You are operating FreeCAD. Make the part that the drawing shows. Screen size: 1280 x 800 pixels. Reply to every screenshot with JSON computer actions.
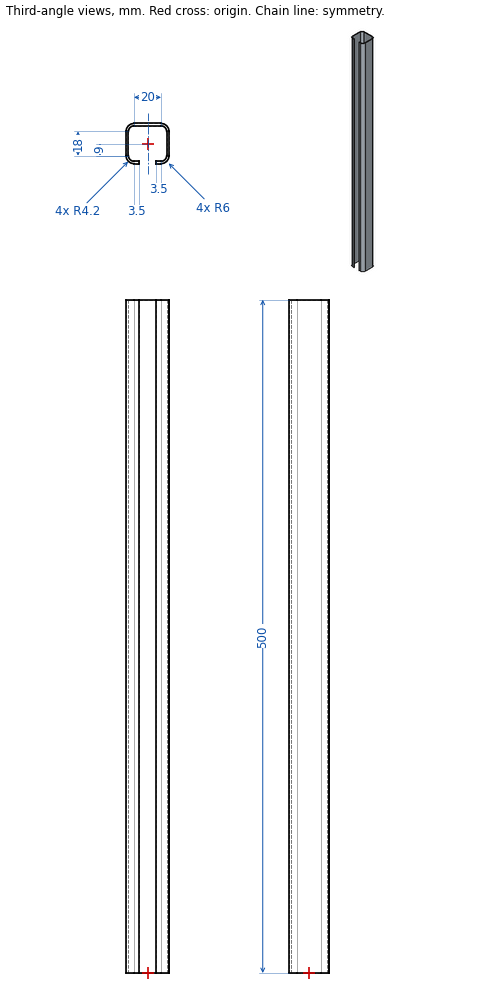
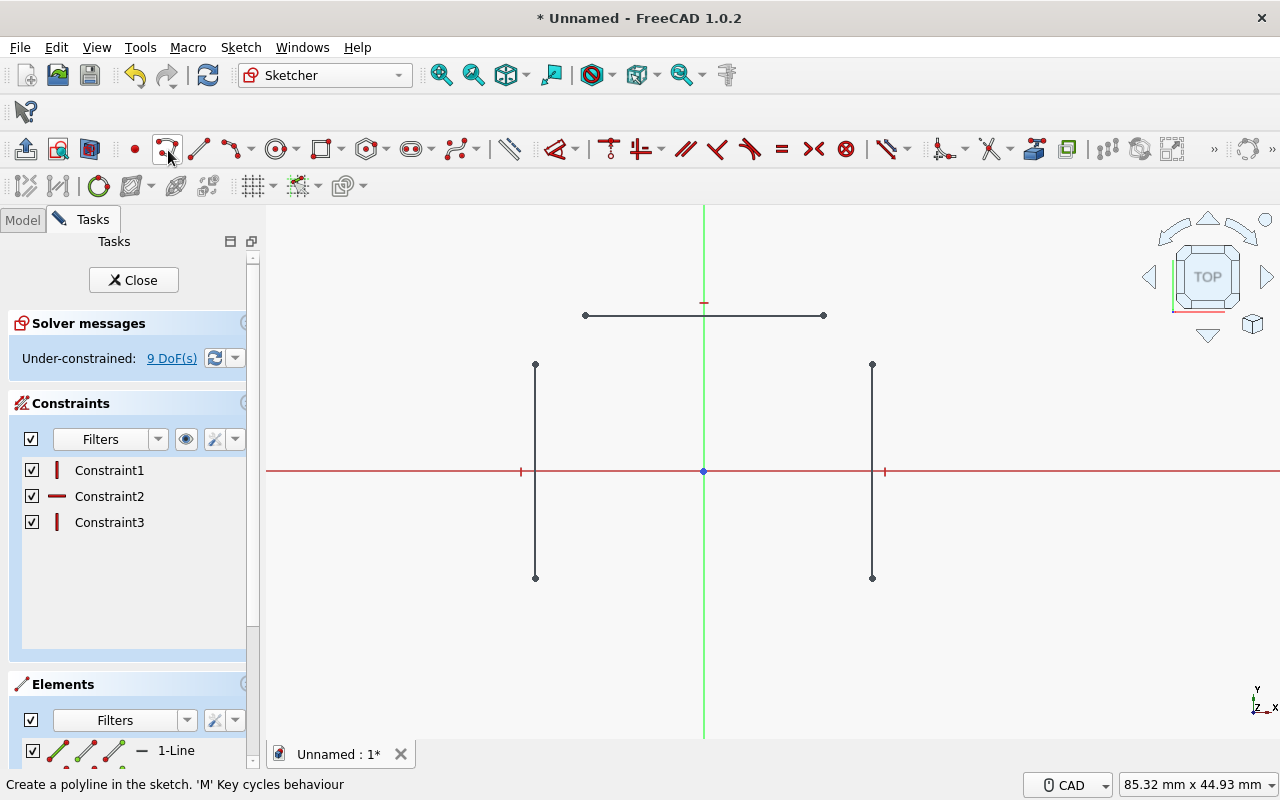
{"action": "left_click", "coordinate": [823, 628]}
{"action": "left_click", "coordinate": [781, 628]}
{"action": "left_click", "coordinate": [781, 650]}
{"action": "left_click", "coordinate": [823, 650]}
{"action": "right_click", "coordinate": [823, 650]}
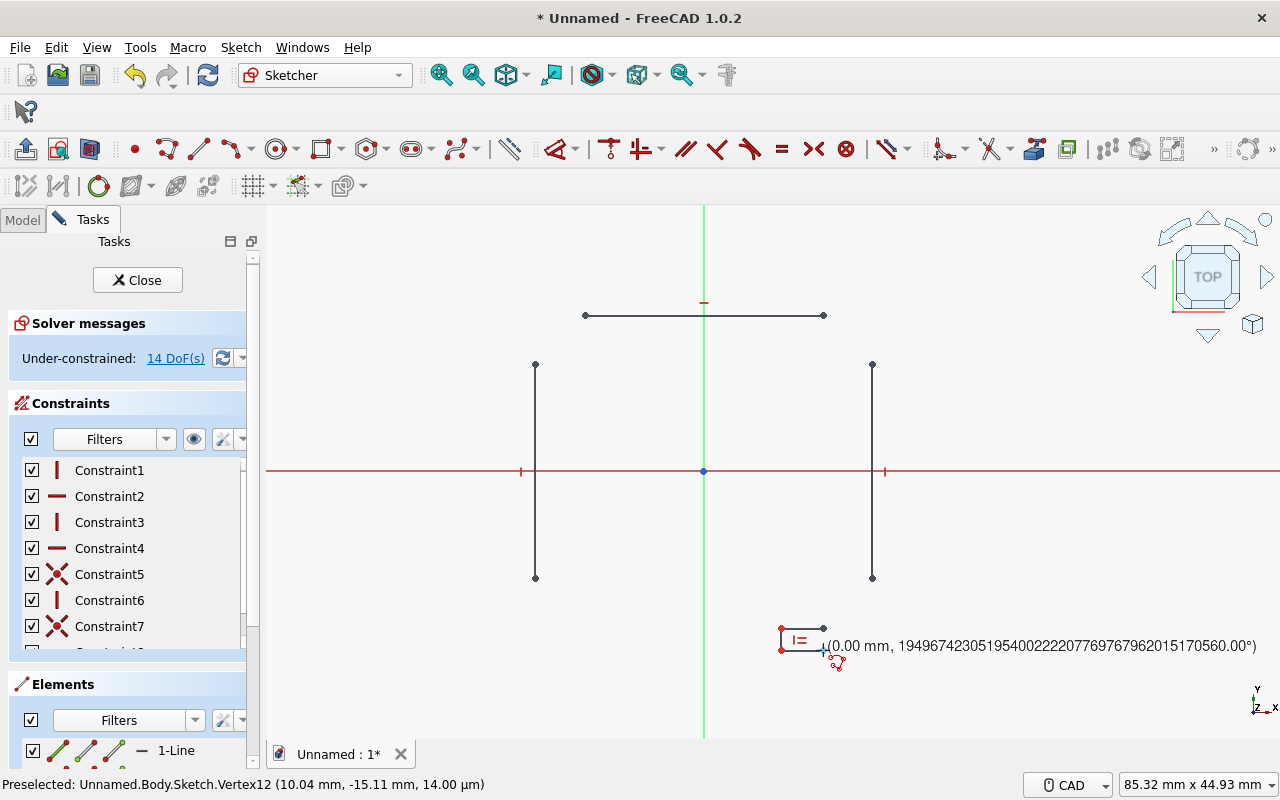
{"action": "left_click", "coordinate": [200, 150]}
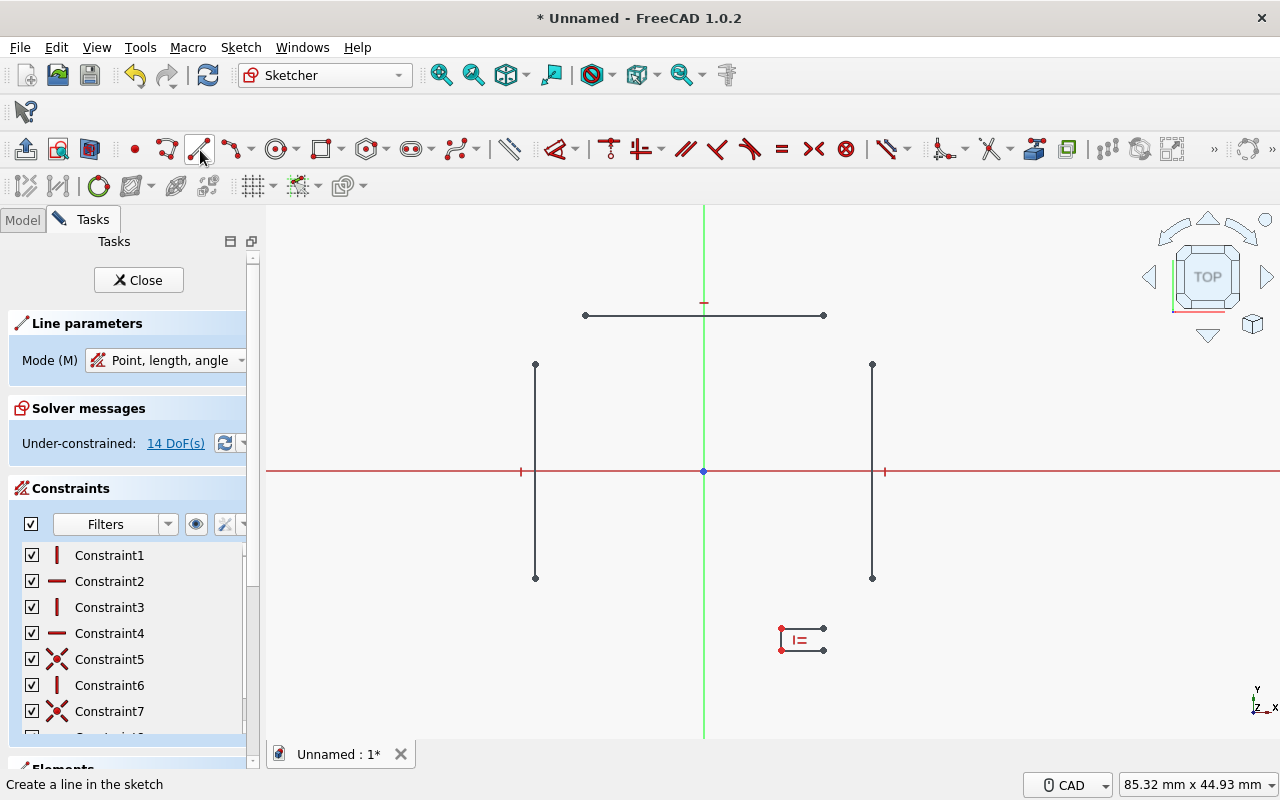
{"action": "left_click", "coordinate": [894, 578]}
{"action": "left_click", "coordinate": [894, 364]}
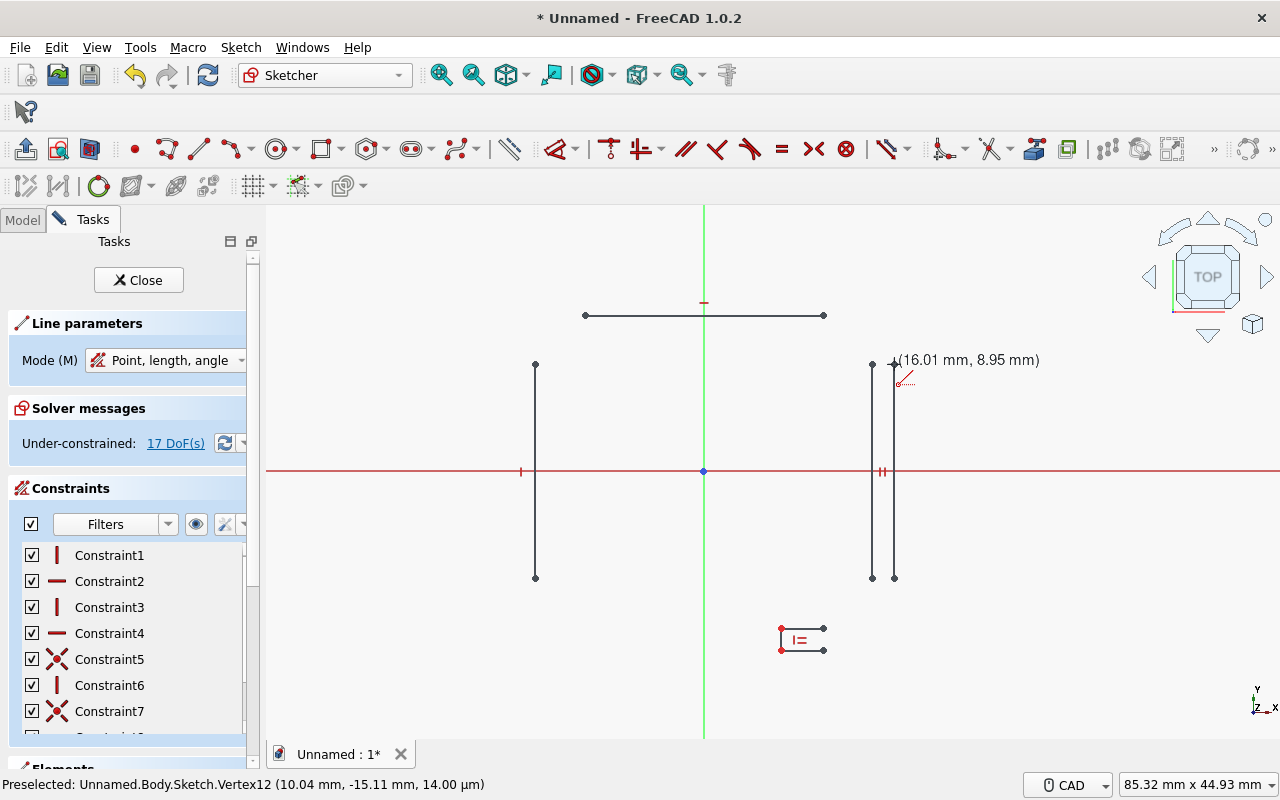
{"action": "left_click", "coordinate": [823, 293]}
{"action": "left_click", "coordinate": [585, 293]}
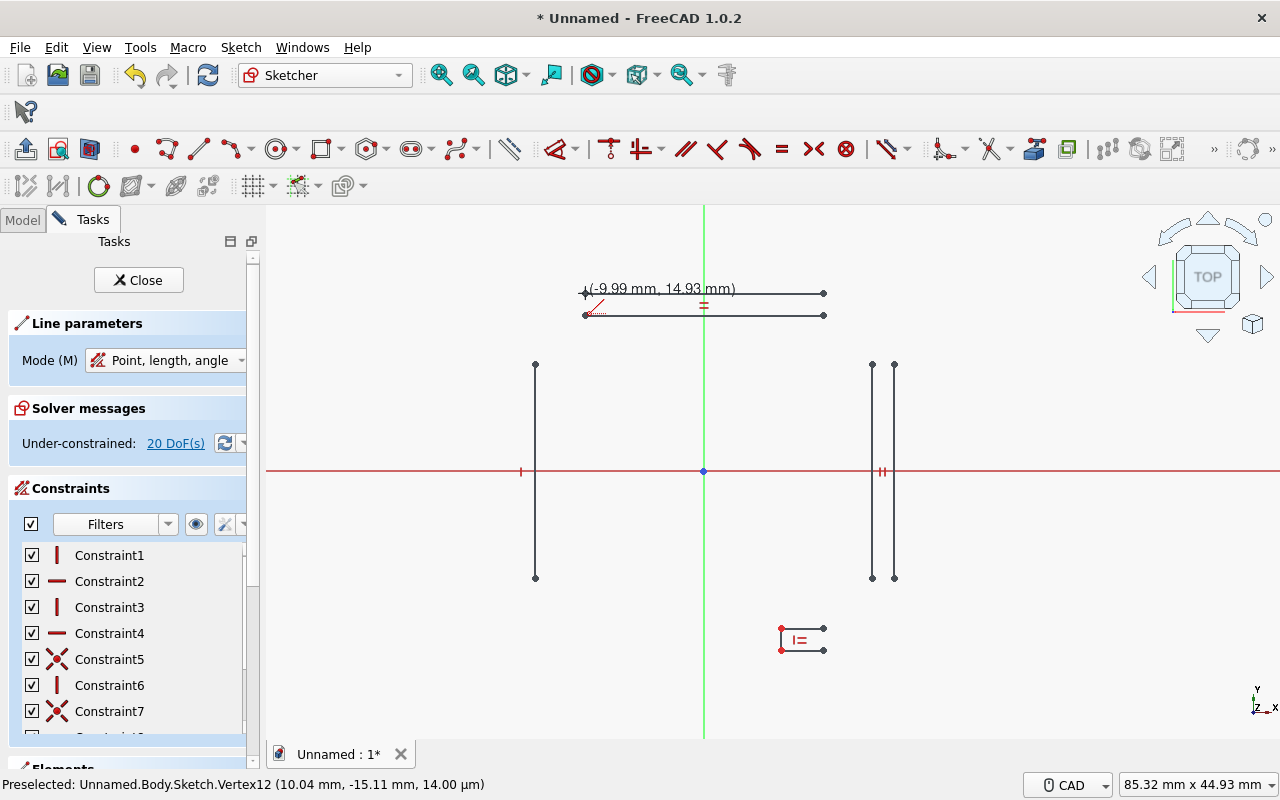
{"action": "left_click", "coordinate": [514, 364]}
{"action": "left_click", "coordinate": [514, 578]}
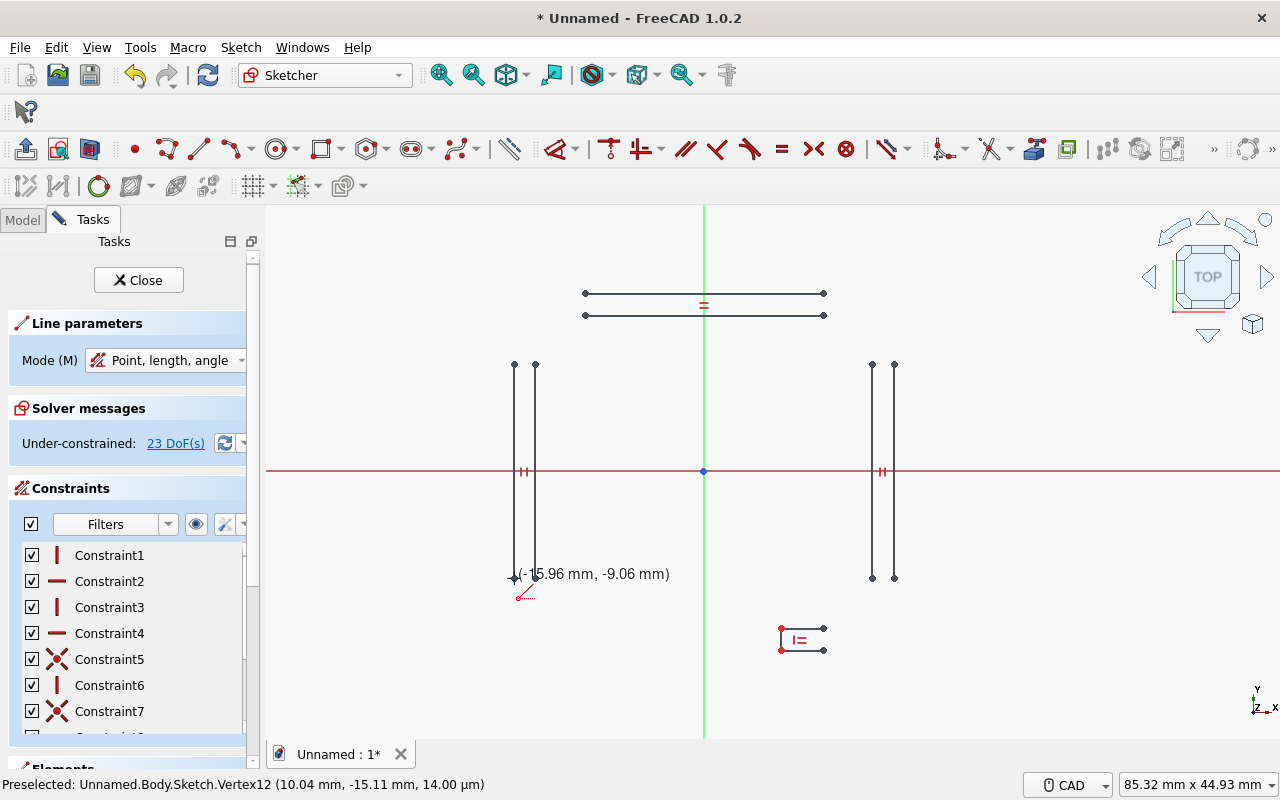
{"action": "left_click", "coordinate": [168, 150]}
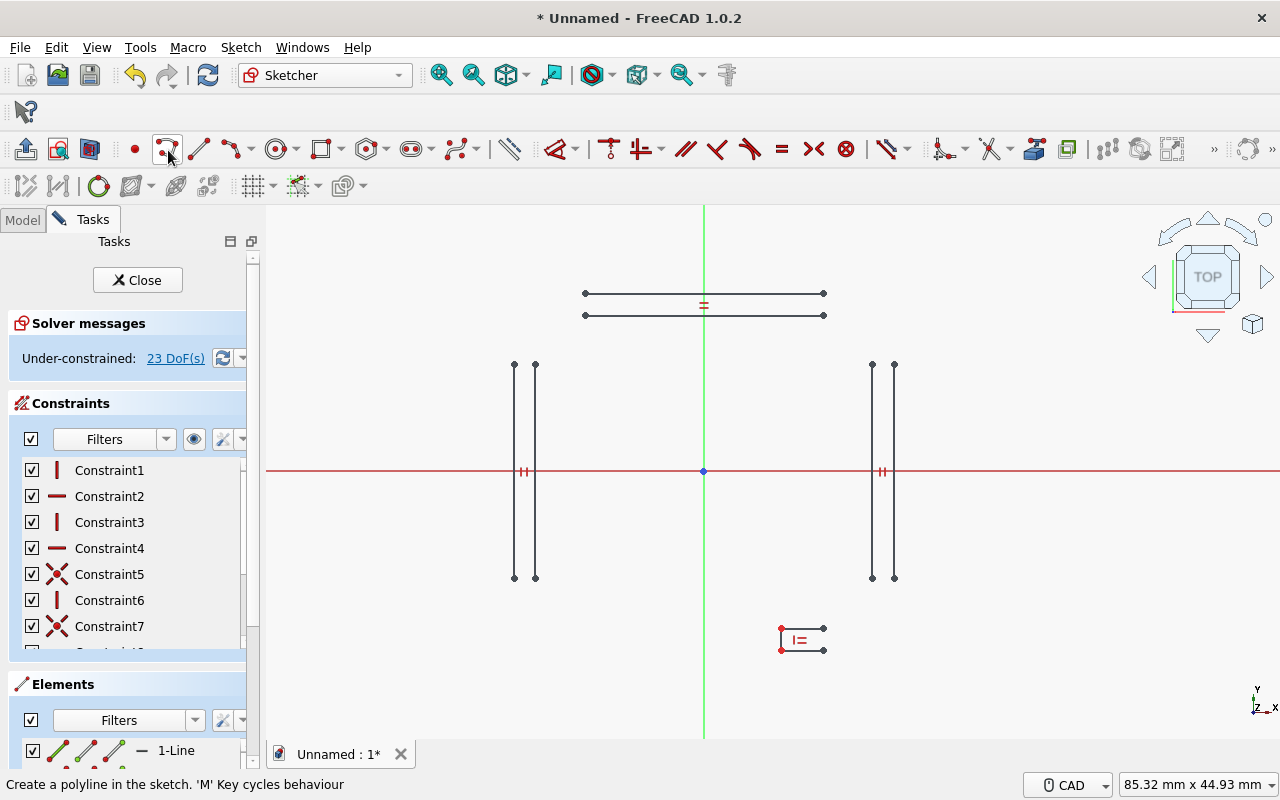
{"action": "left_click", "coordinate": [585, 650]}
{"action": "left_click", "coordinate": [626, 650]}
{"action": "left_click", "coordinate": [626, 628]}
{"action": "left_click", "coordinate": [585, 628]}
{"action": "right_click", "coordinate": [585, 628]}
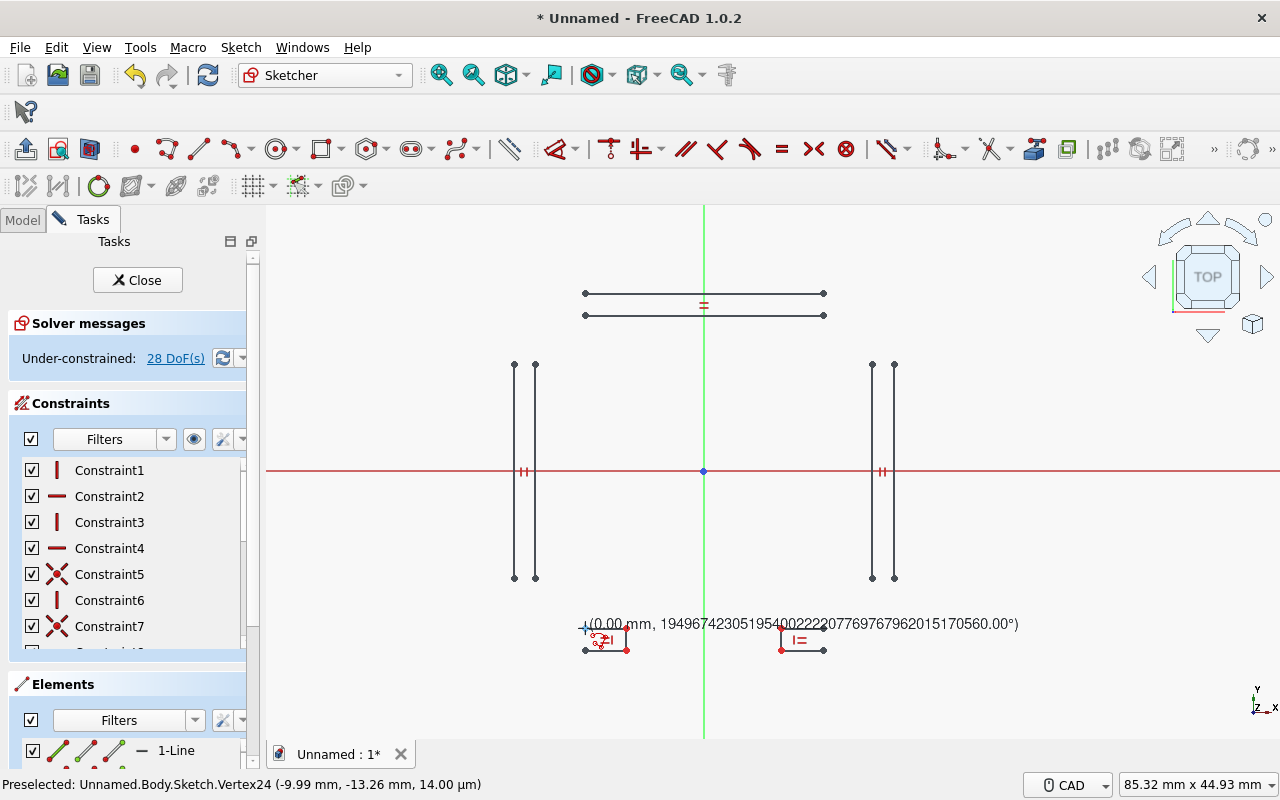
{"action": "left_click", "coordinate": [232, 150]}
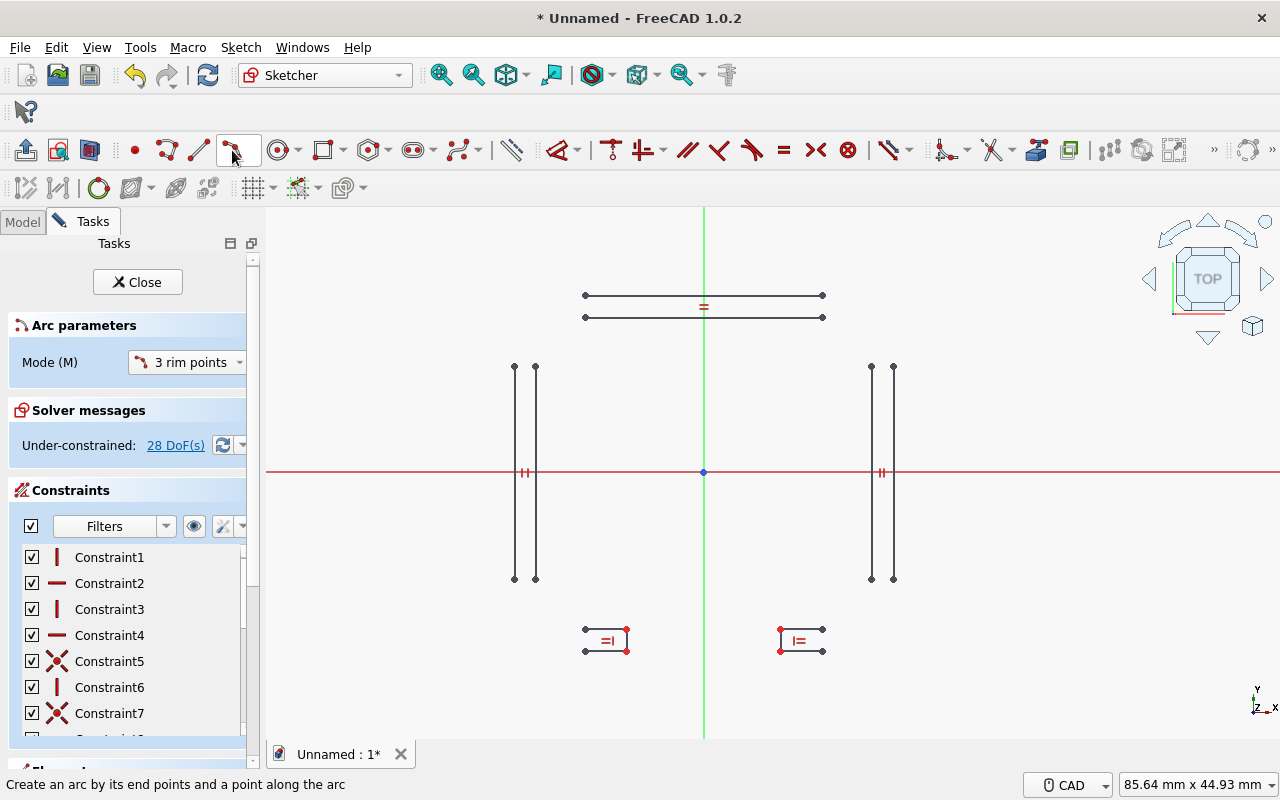
{"action": "left_click", "coordinate": [536, 366]}
{"action": "left_click", "coordinate": [586, 318]}
{"action": "left_click", "coordinate": [550, 331]}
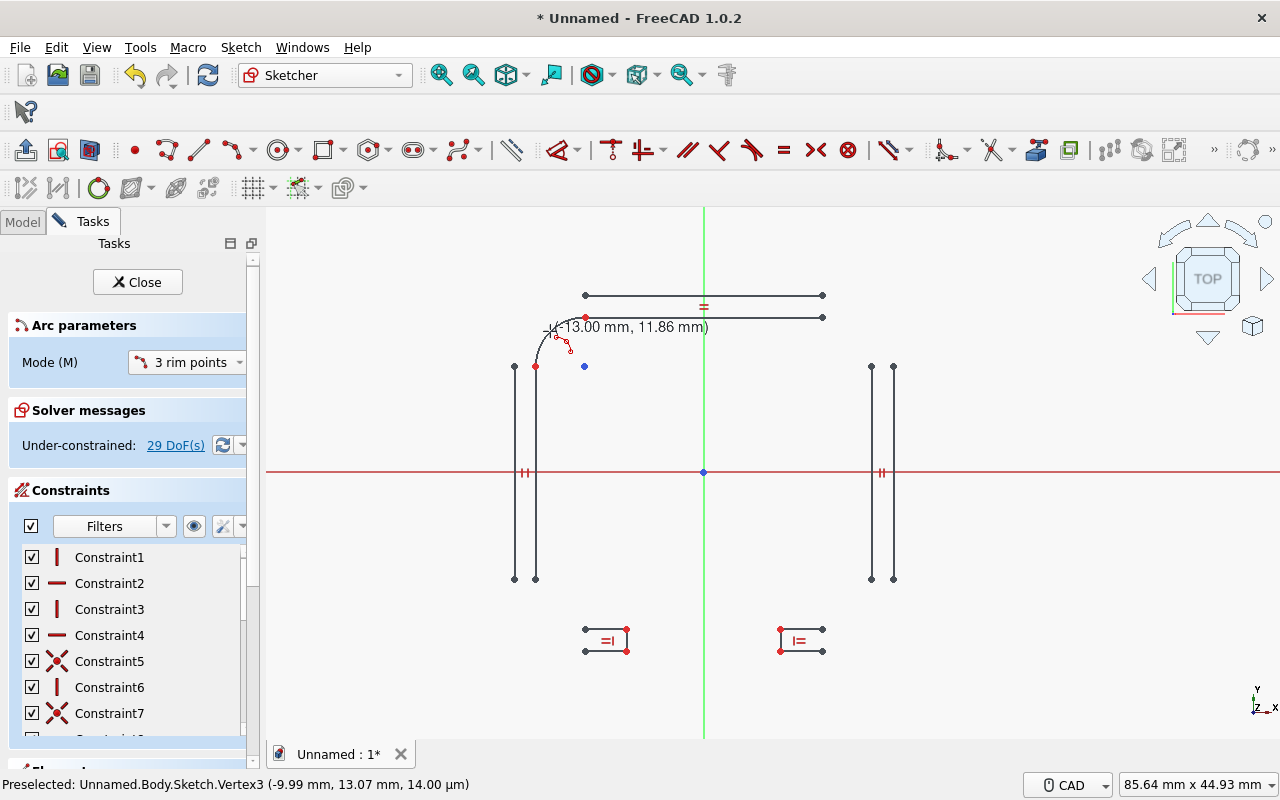
{"action": "left_click", "coordinate": [823, 318]}
{"action": "left_click", "coordinate": [872, 366]}
{"action": "left_click", "coordinate": [858, 331]}